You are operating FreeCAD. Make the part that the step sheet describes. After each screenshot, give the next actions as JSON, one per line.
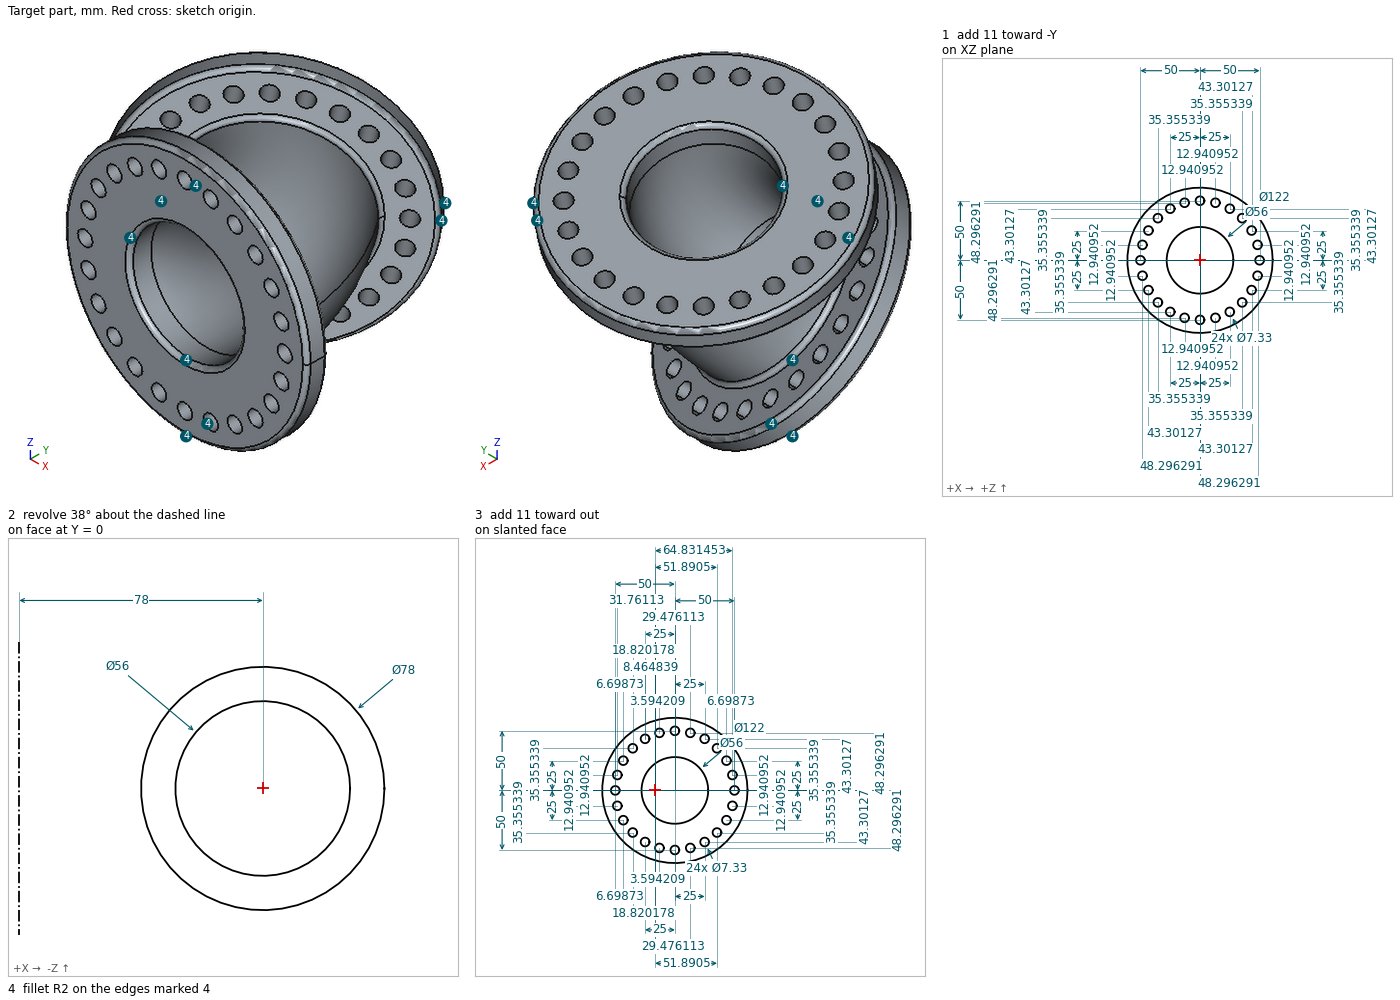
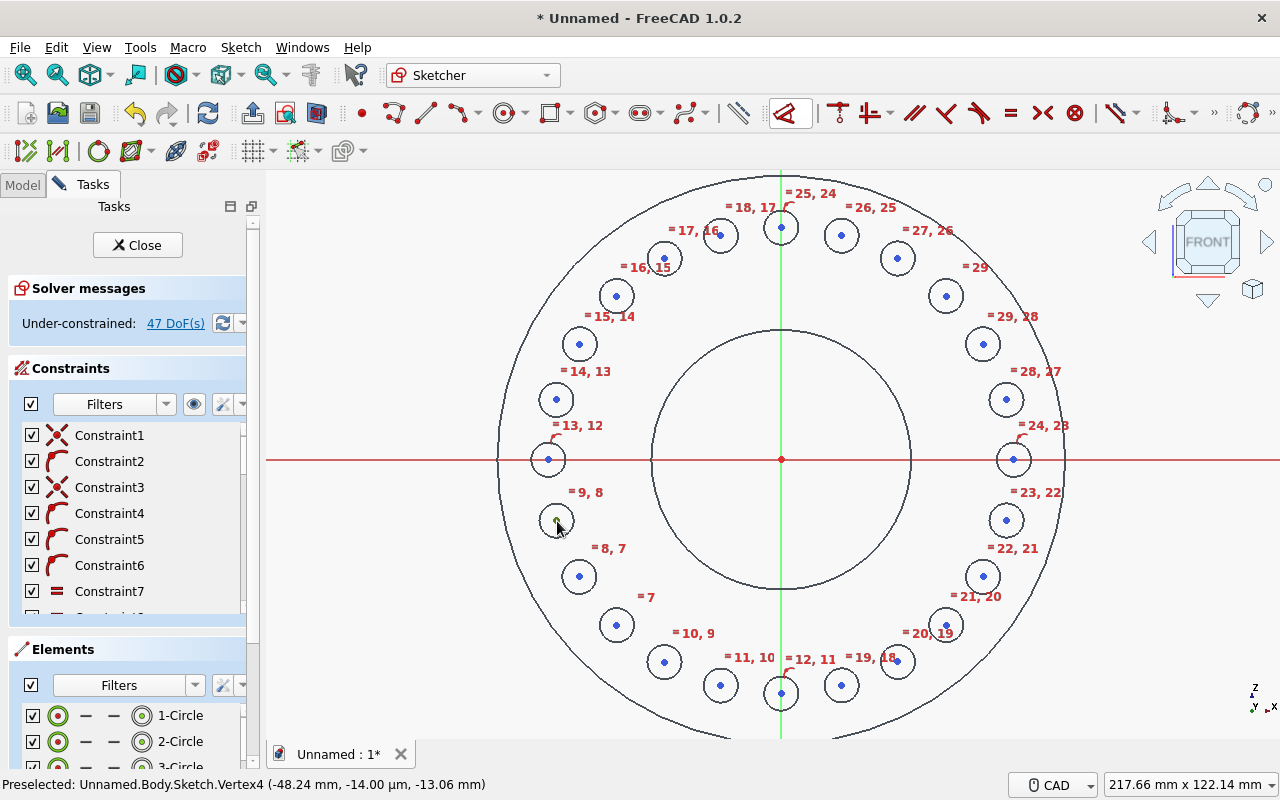
{"action": "left_click", "coordinate": [556, 400]}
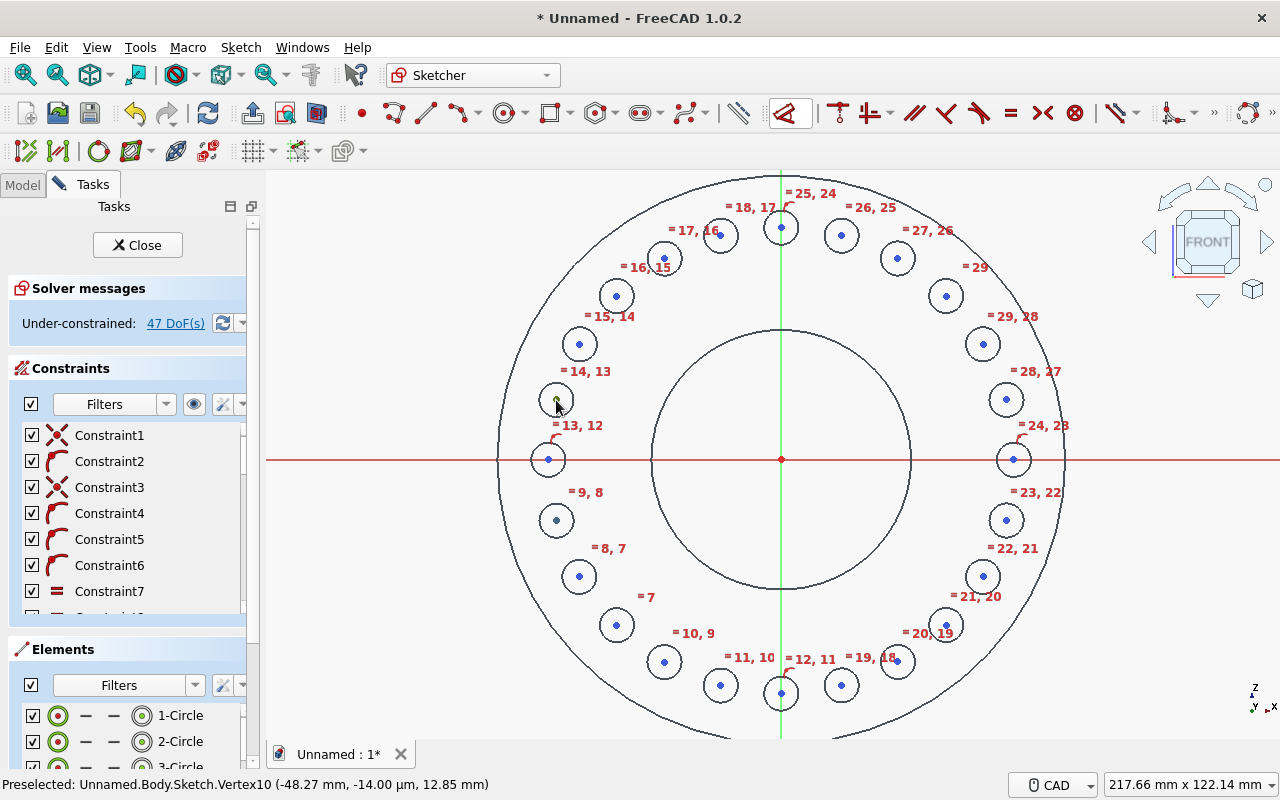
{"action": "key", "text": "v"}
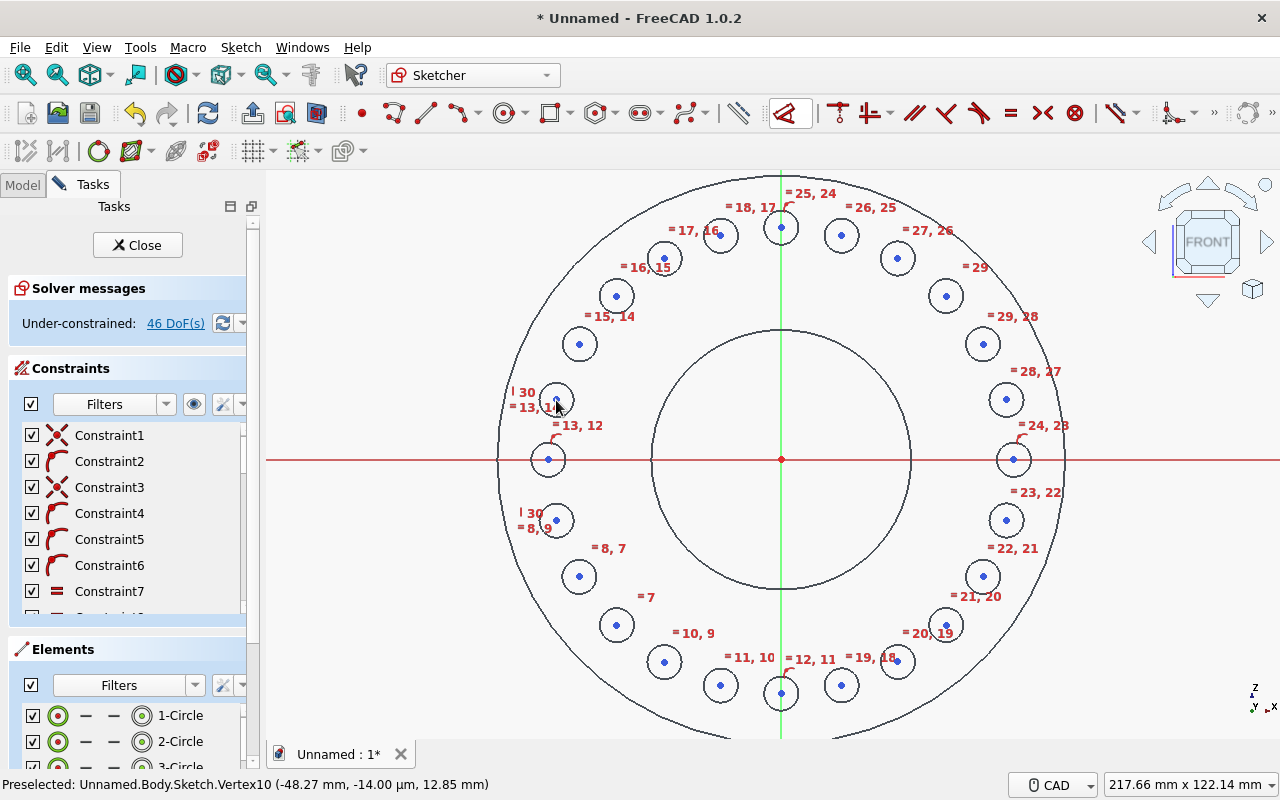
{"action": "left_click", "coordinate": [579, 577]}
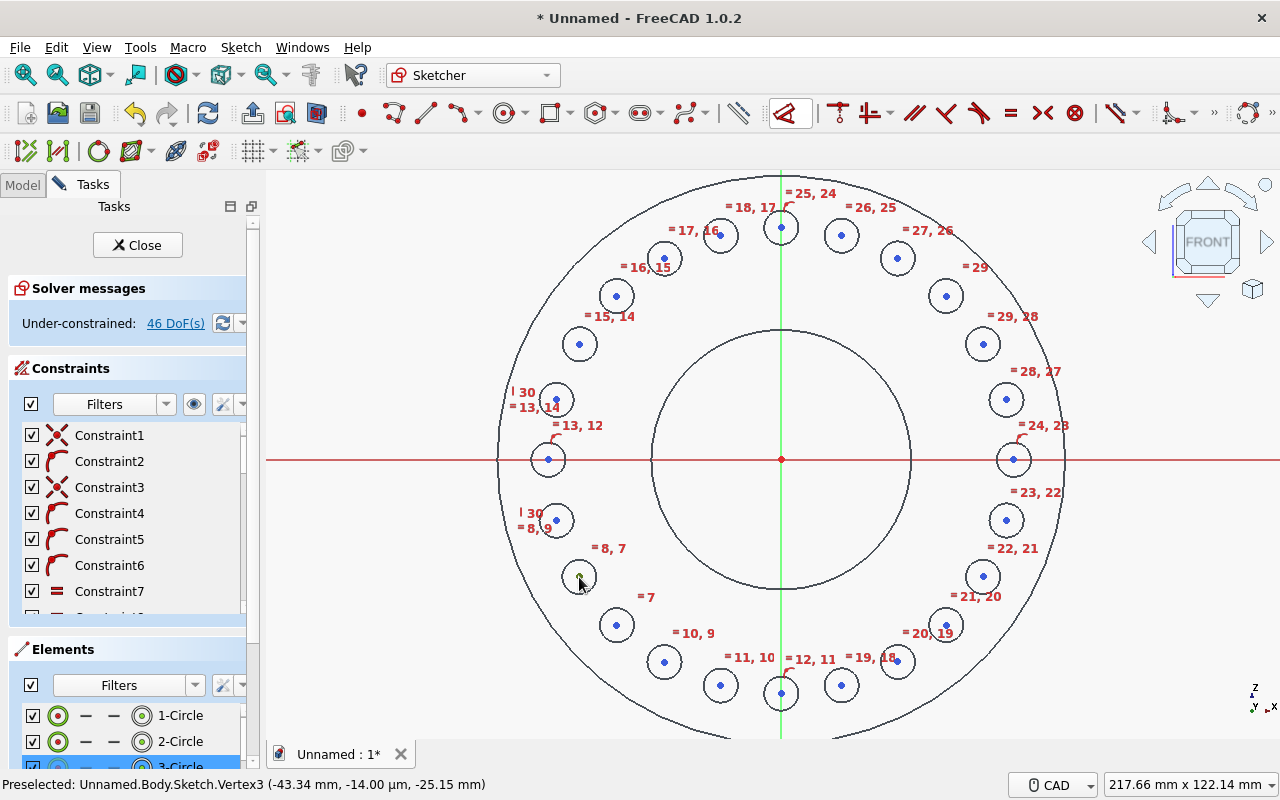
{"action": "left_click", "coordinate": [580, 344]}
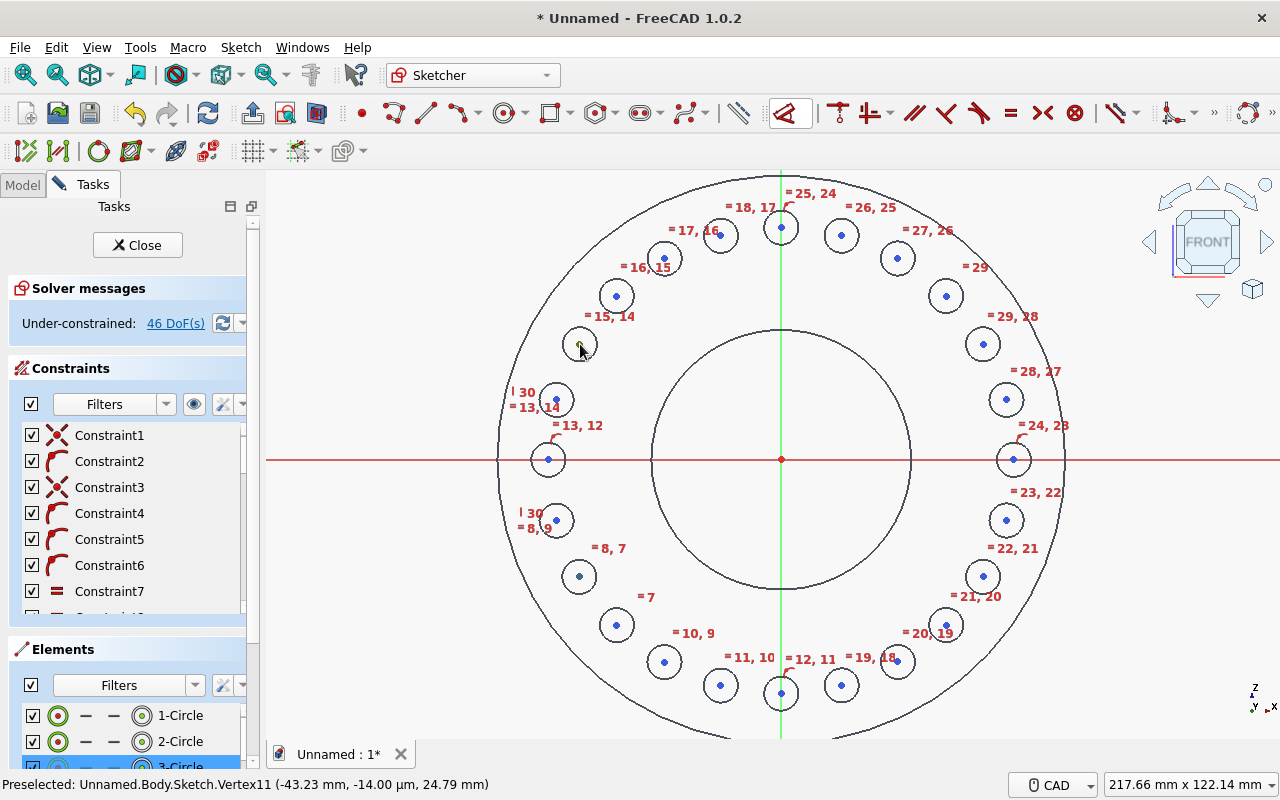
{"action": "left_click", "coordinate": [892, 114]}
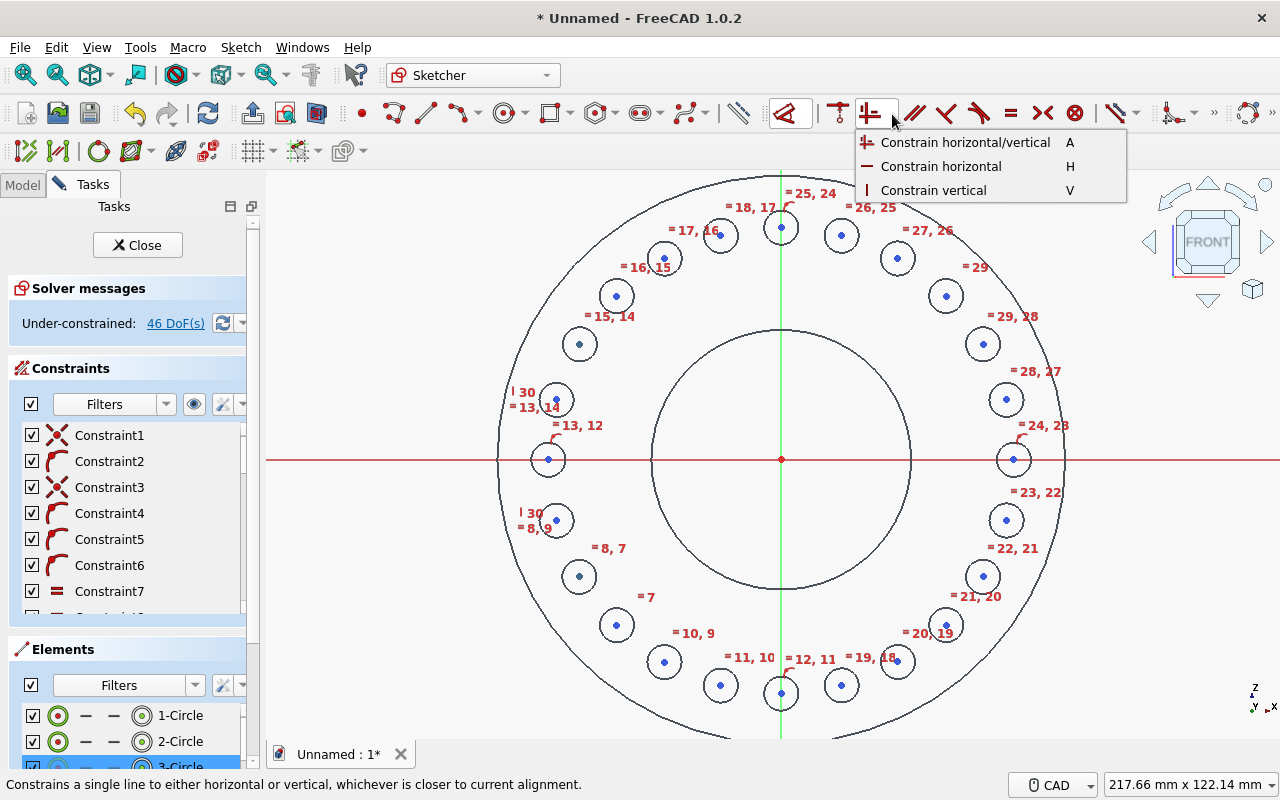
{"action": "left_click", "coordinate": [991, 190]}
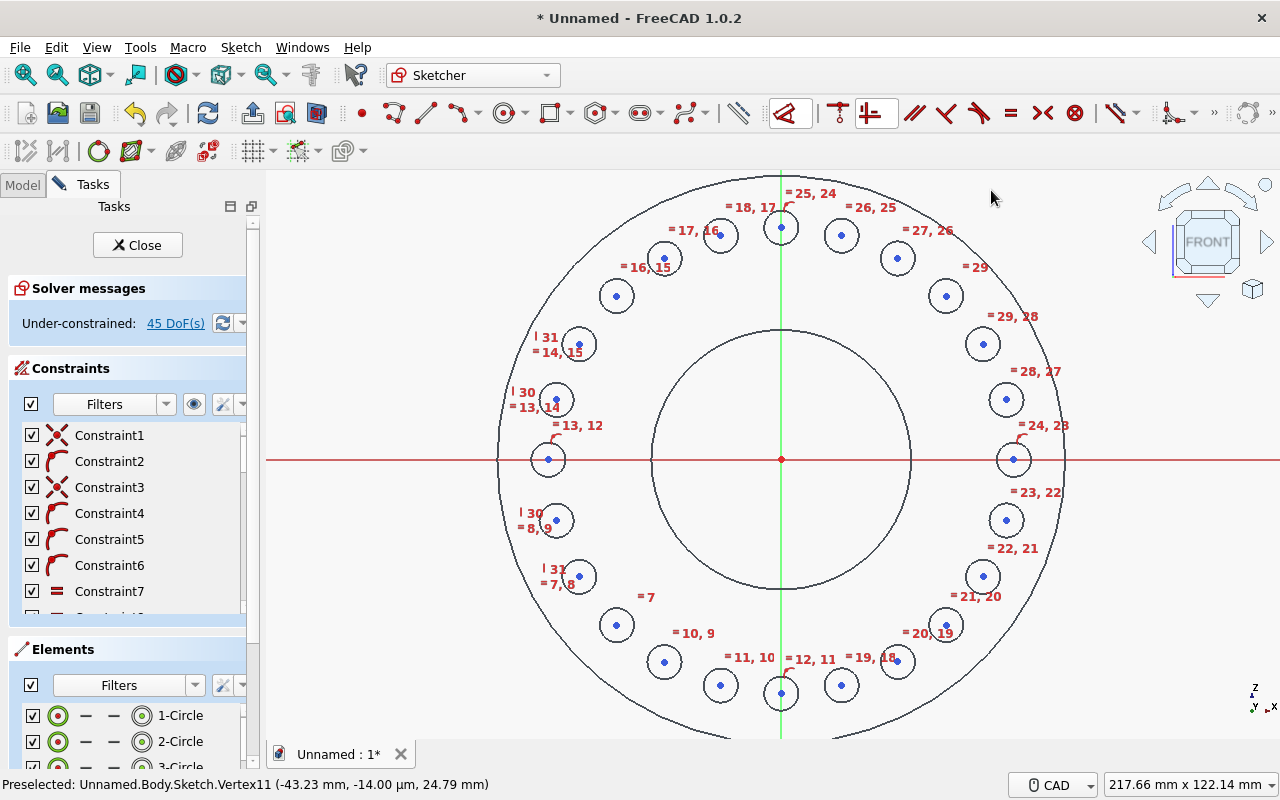
{"action": "left_click", "coordinate": [721, 686]}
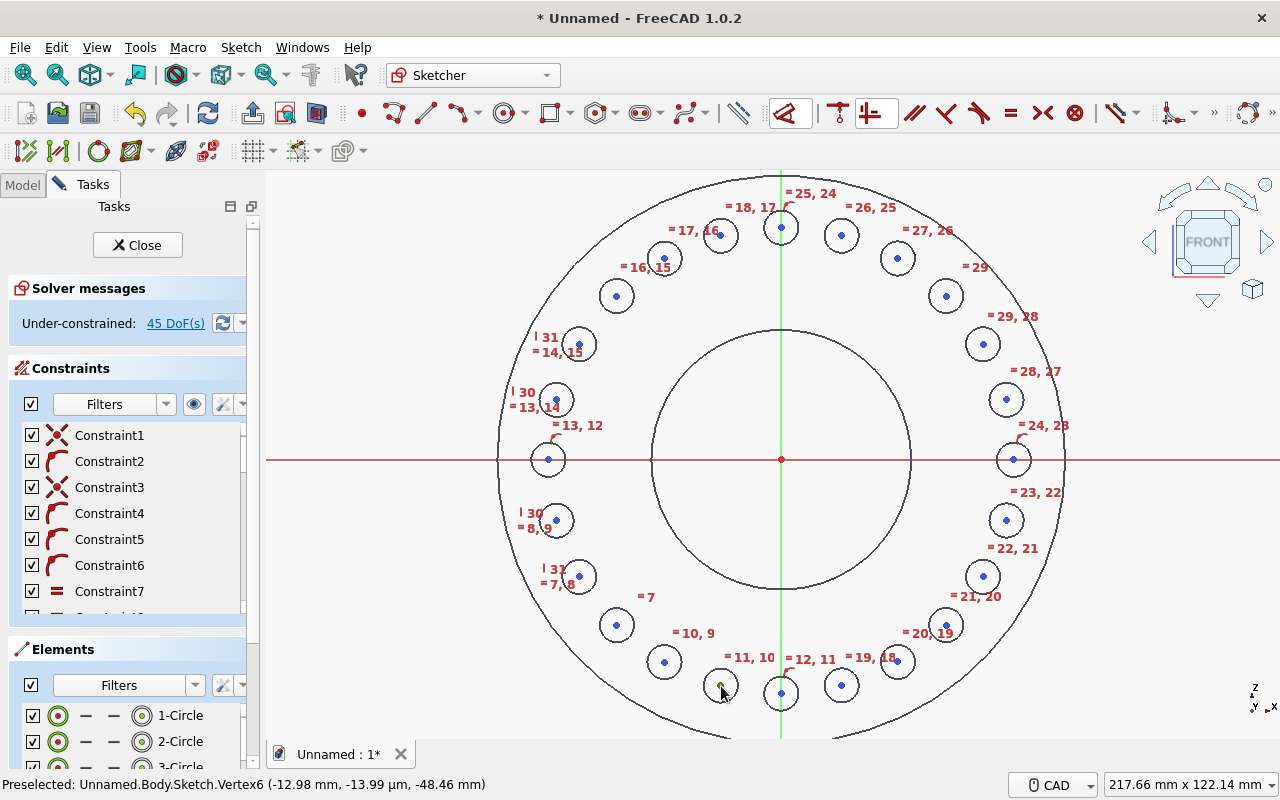
{"action": "left_click", "coordinate": [842, 685]}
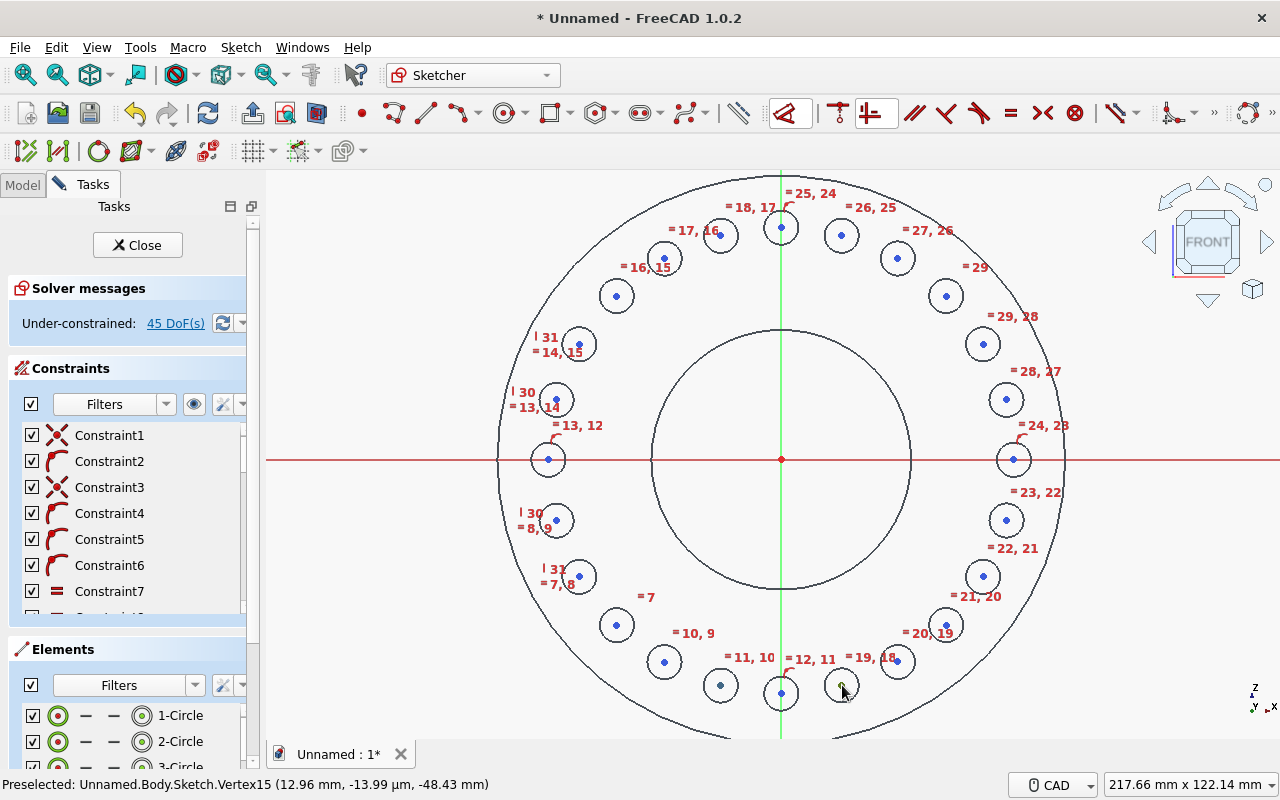
{"action": "key", "text": "h"}